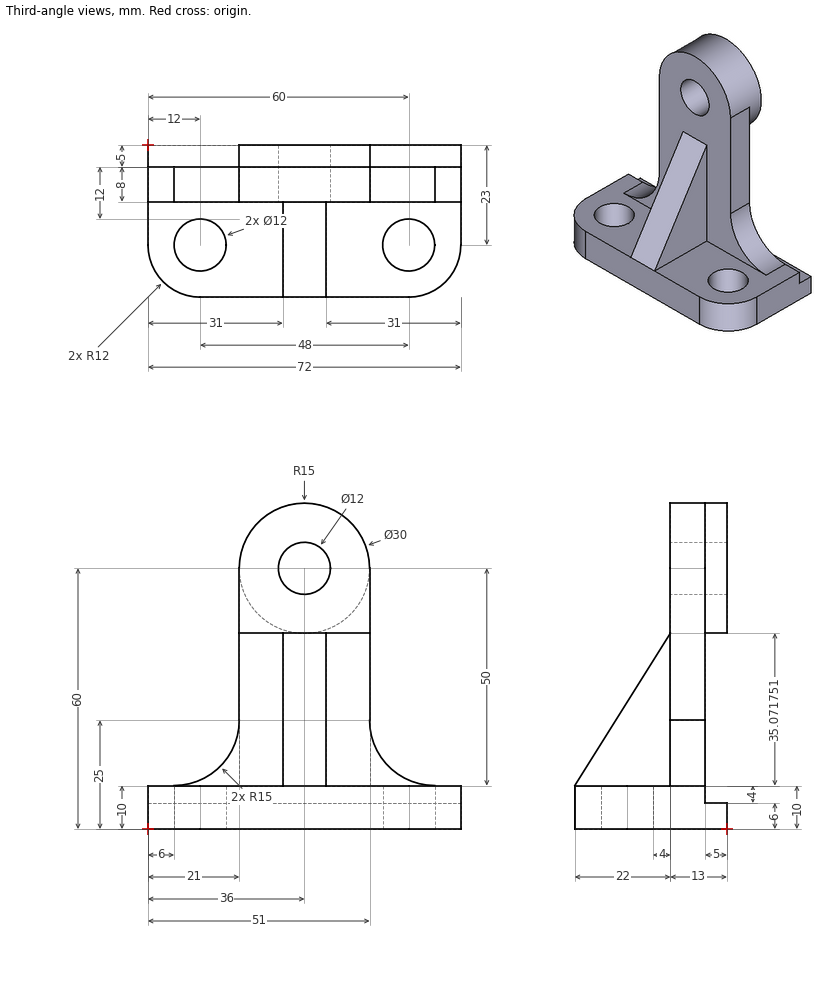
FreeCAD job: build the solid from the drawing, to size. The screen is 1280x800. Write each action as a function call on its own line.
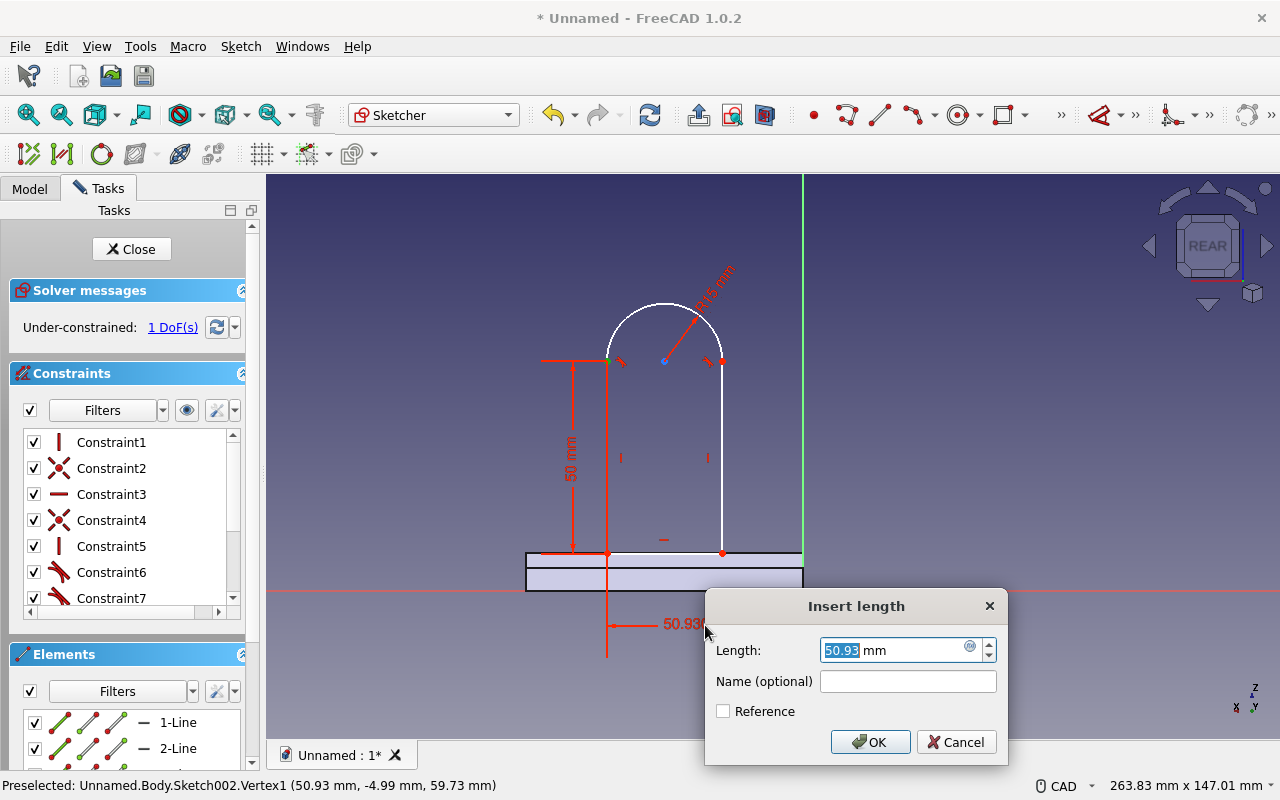
text(51)
key(Return)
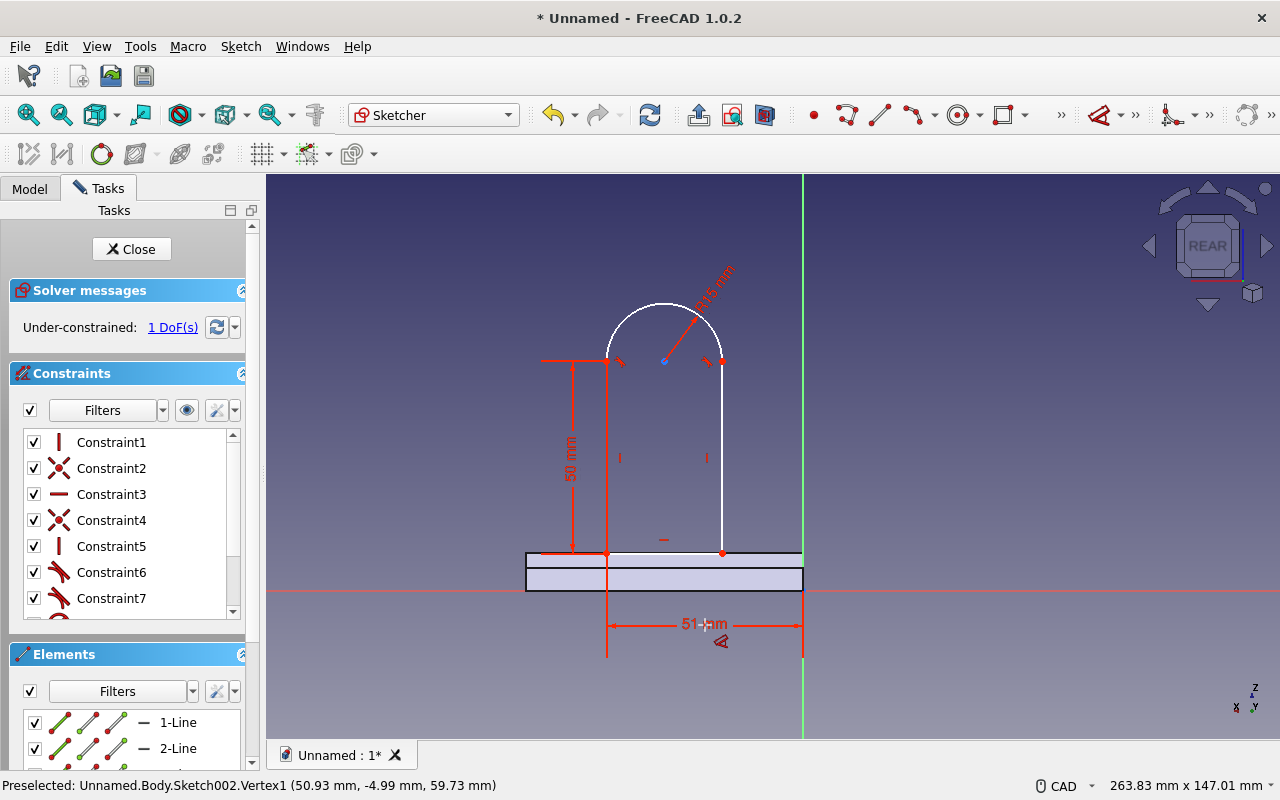
click(607, 361)
click(837, 476)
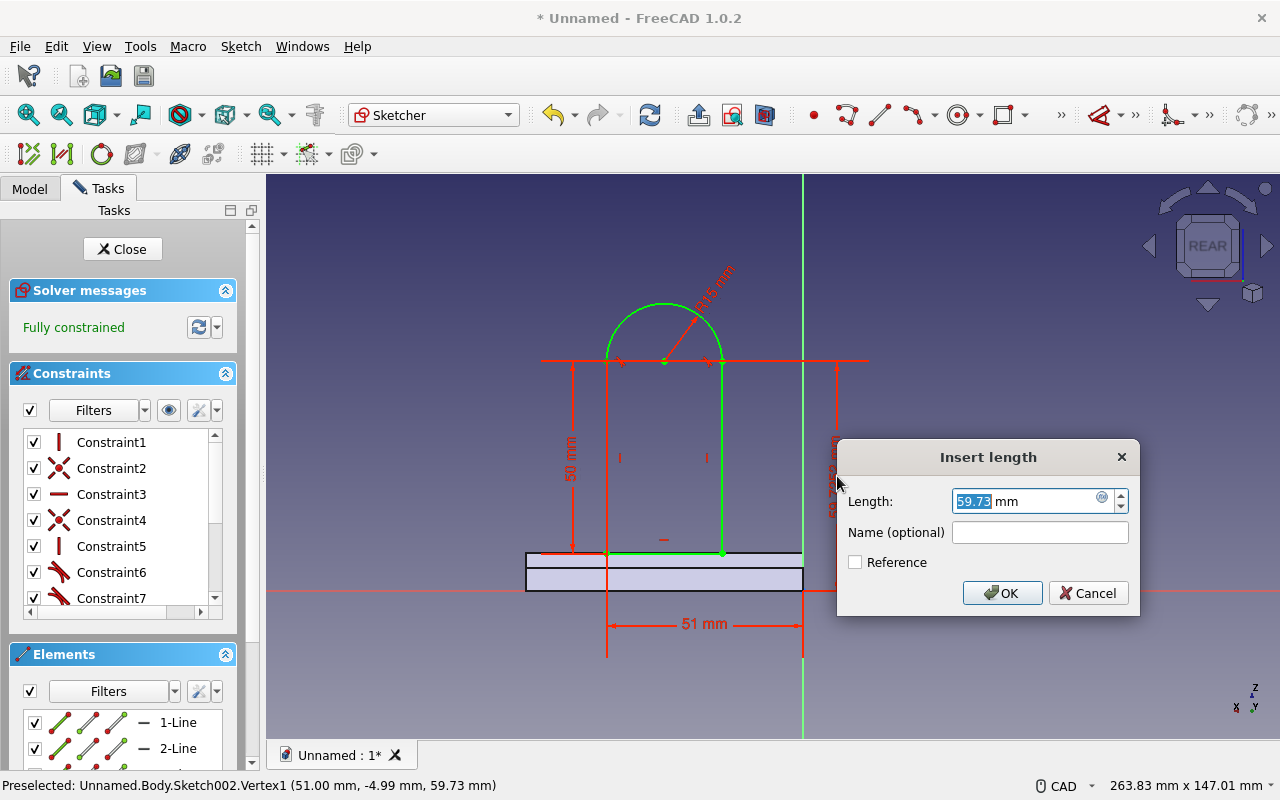
text(60)
key(Return)
key(Escape)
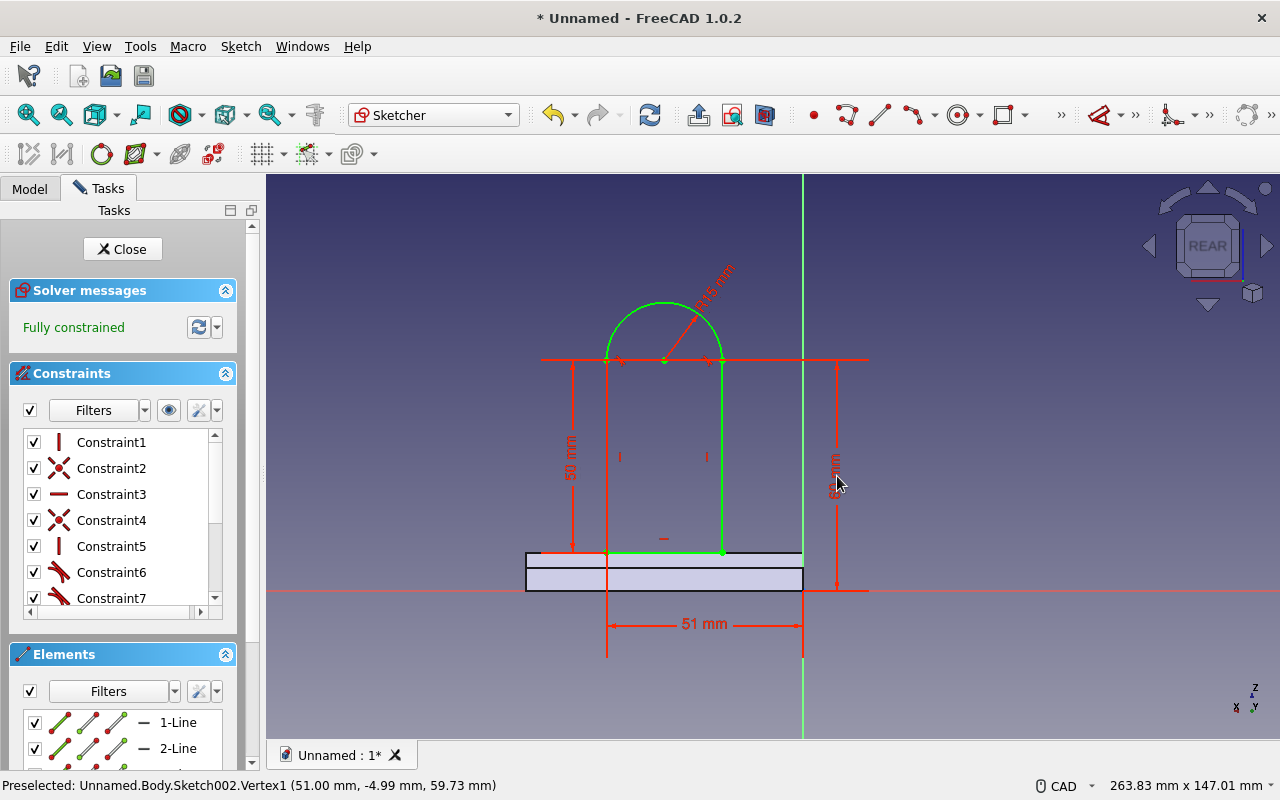
click(123, 249)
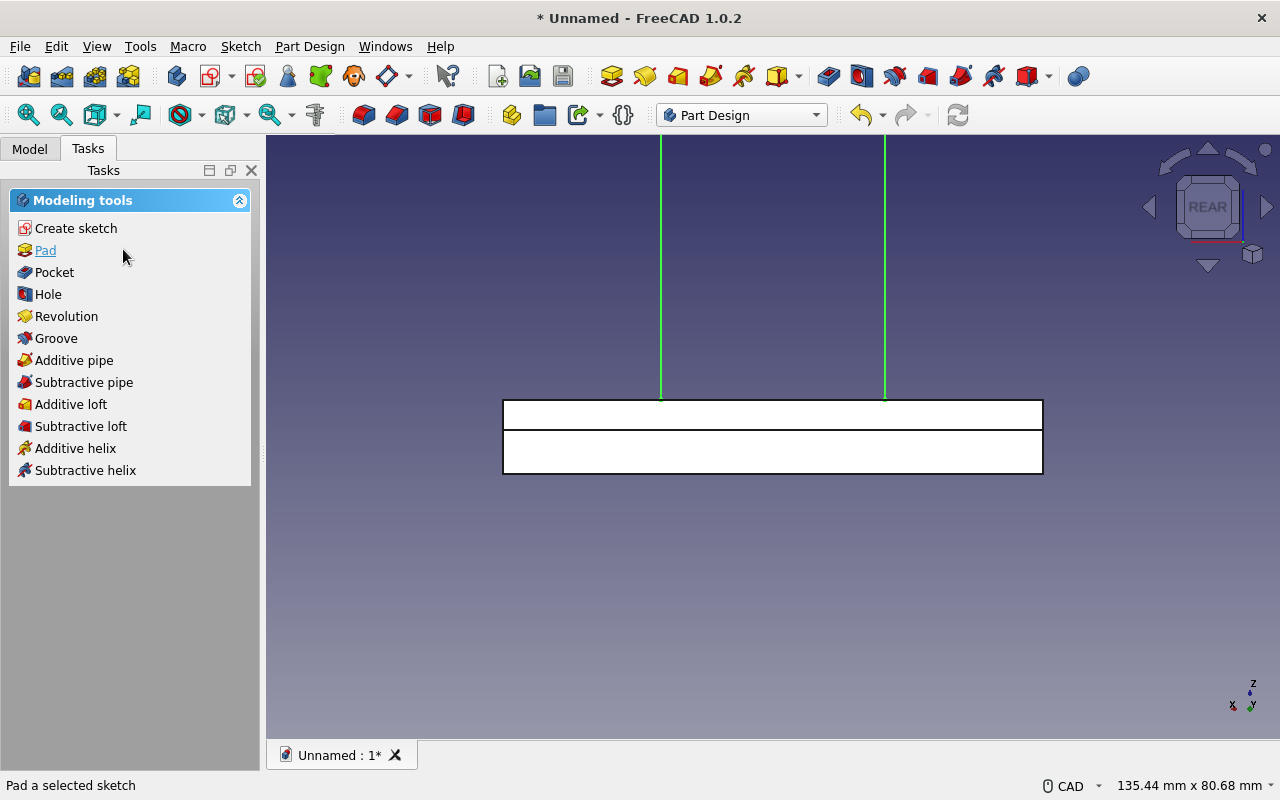
click(612, 76)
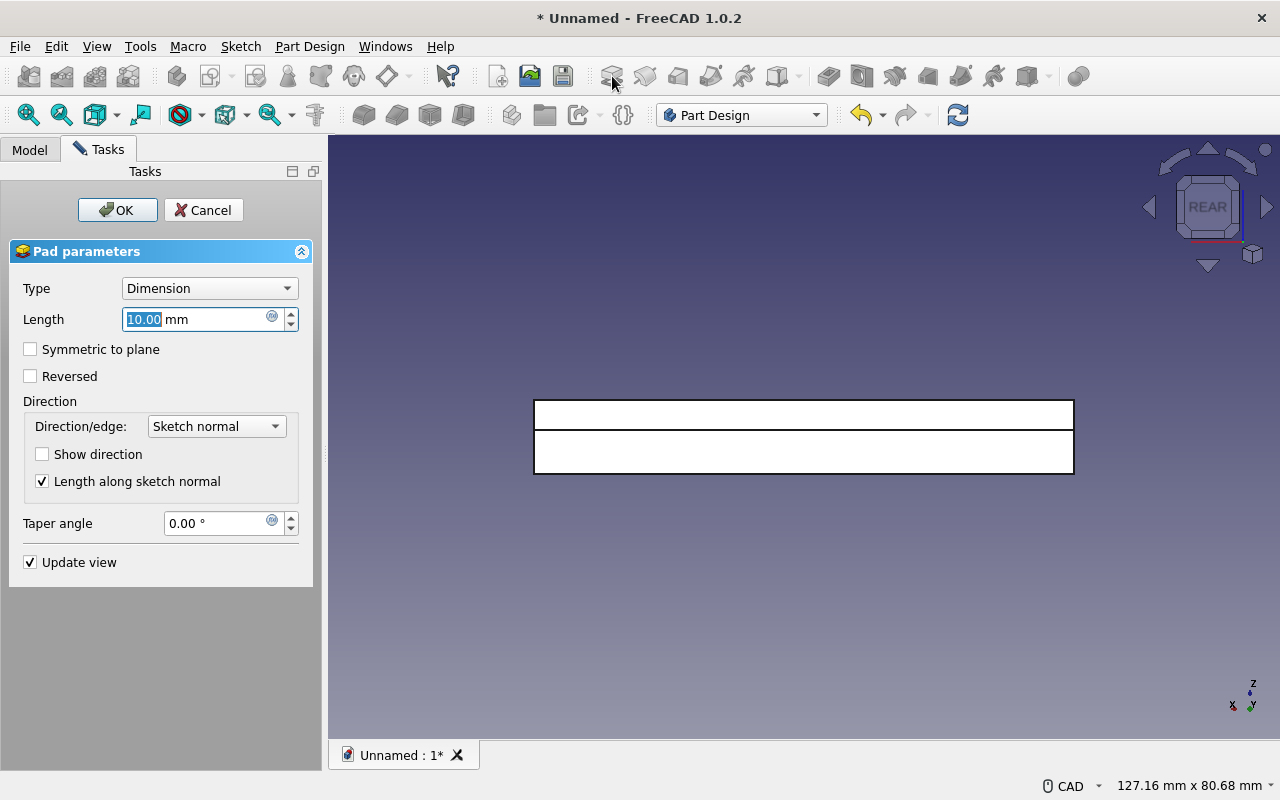
text(12)
key(Tab)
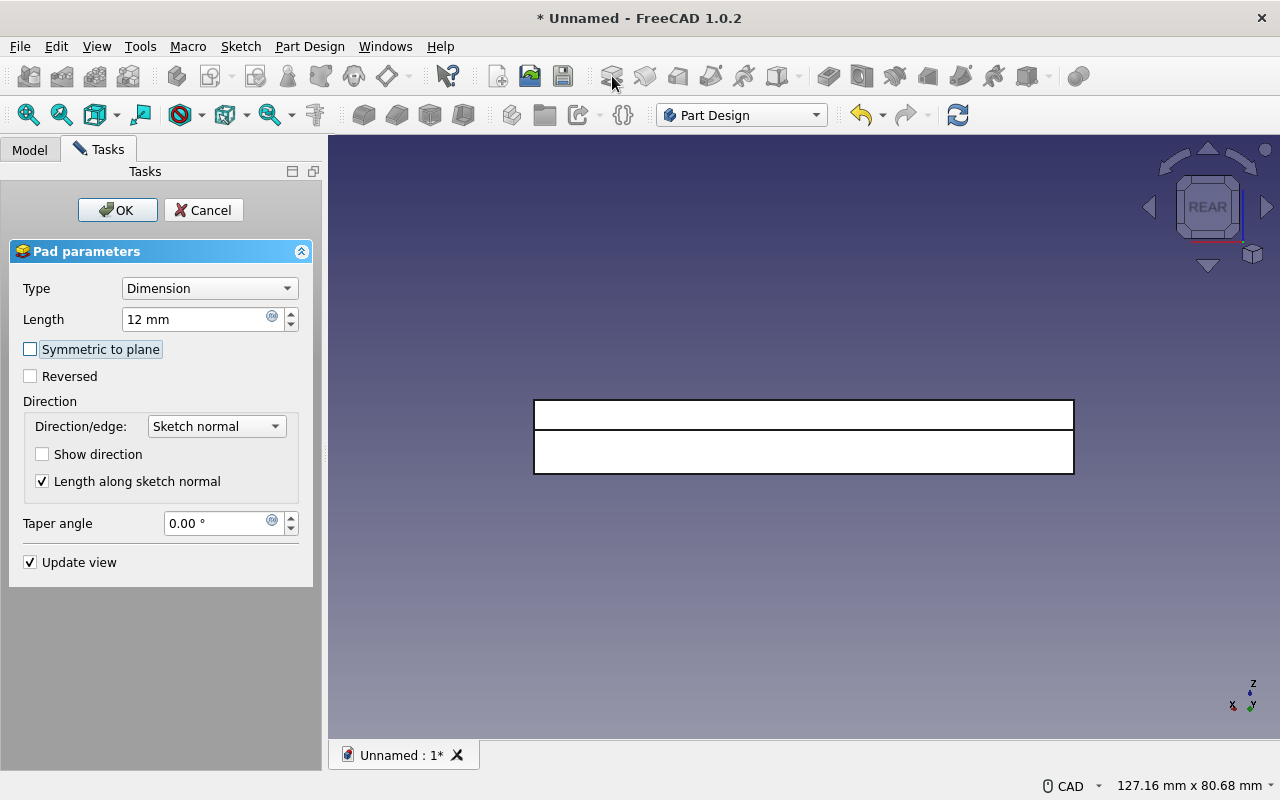
click(31, 376)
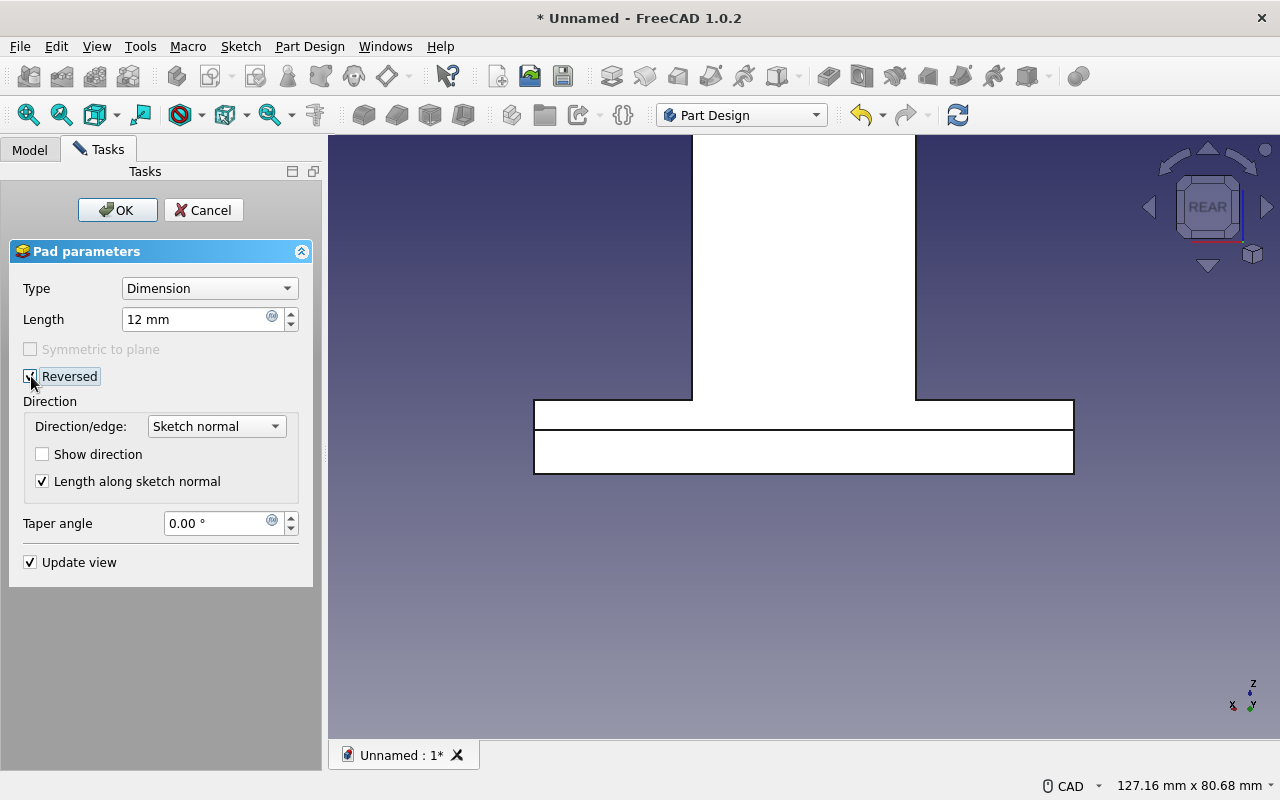
click(118, 210)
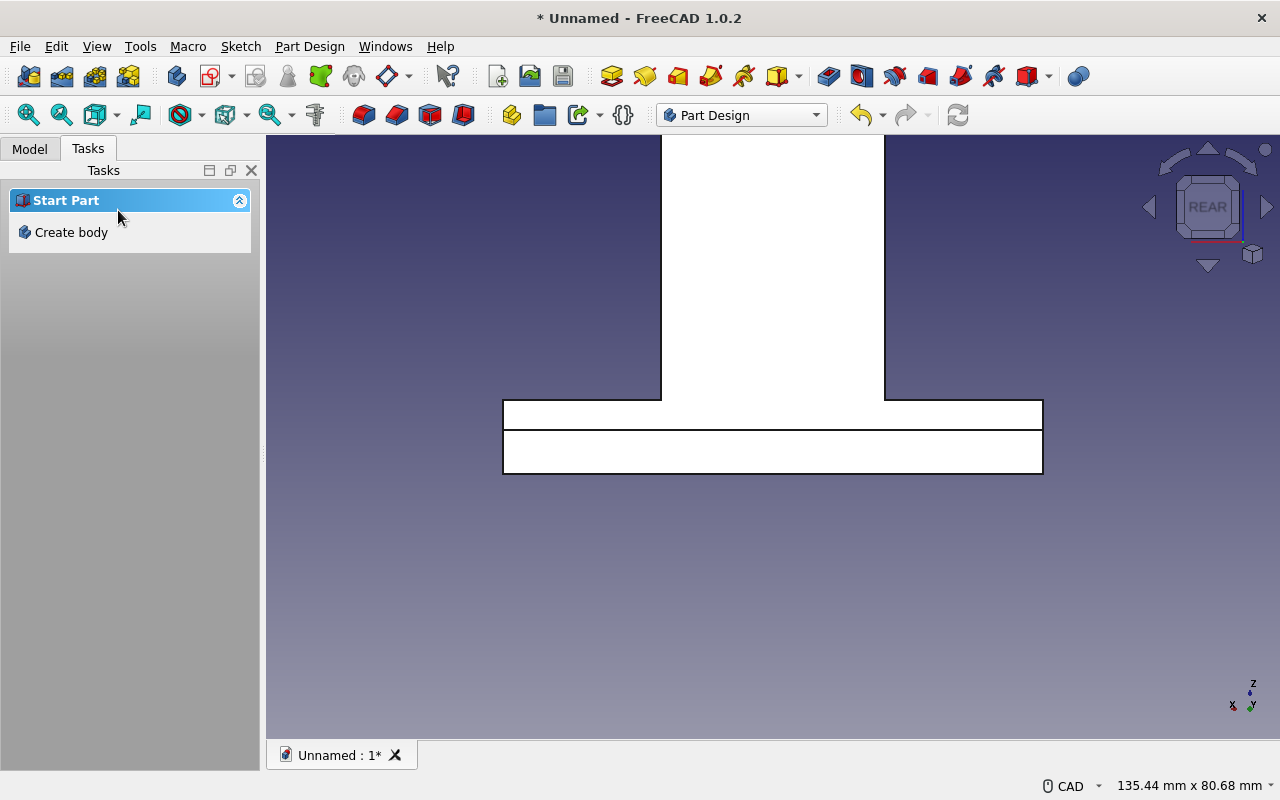
click(29, 116)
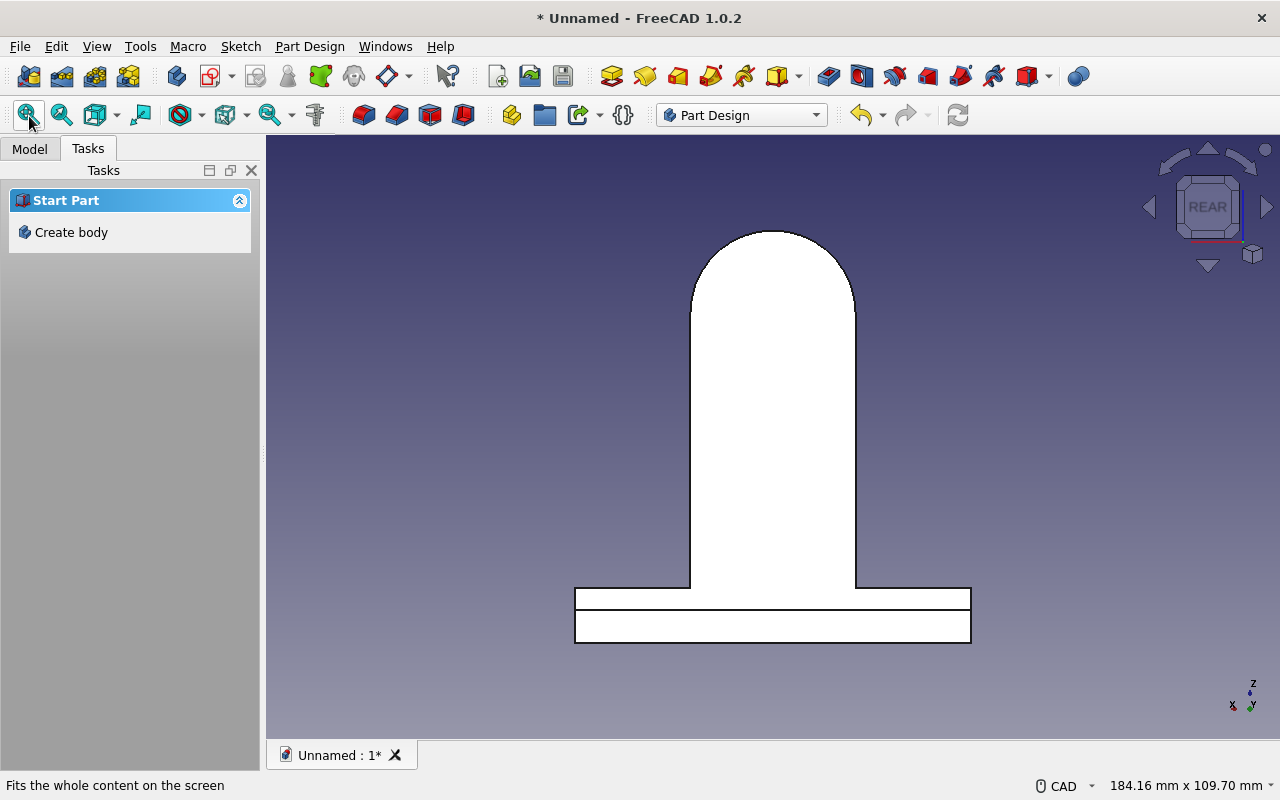
click(603, 626)